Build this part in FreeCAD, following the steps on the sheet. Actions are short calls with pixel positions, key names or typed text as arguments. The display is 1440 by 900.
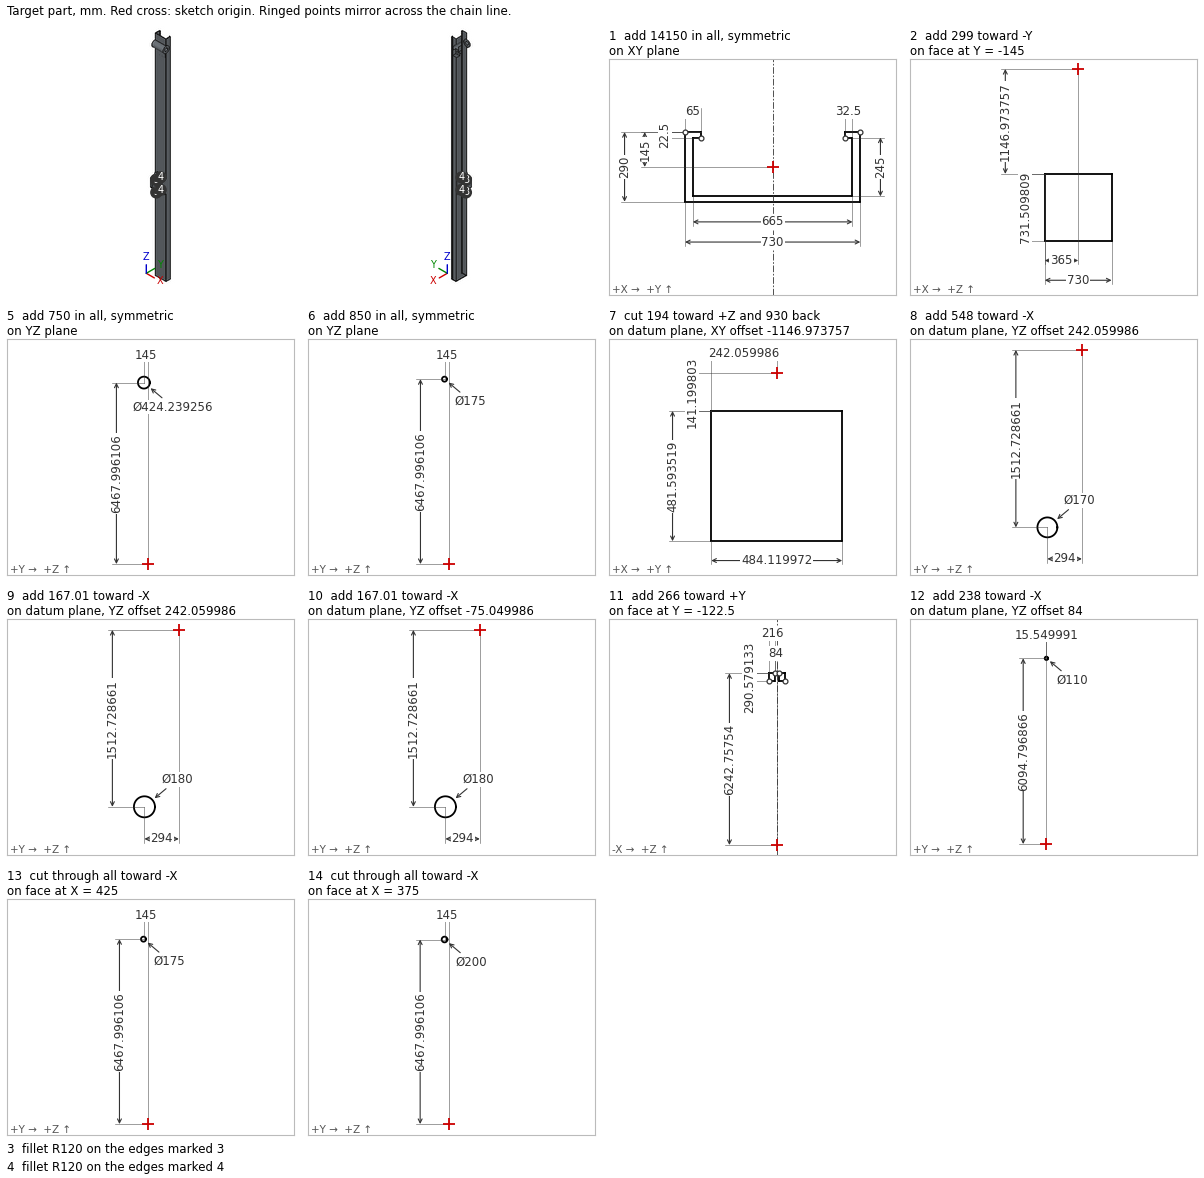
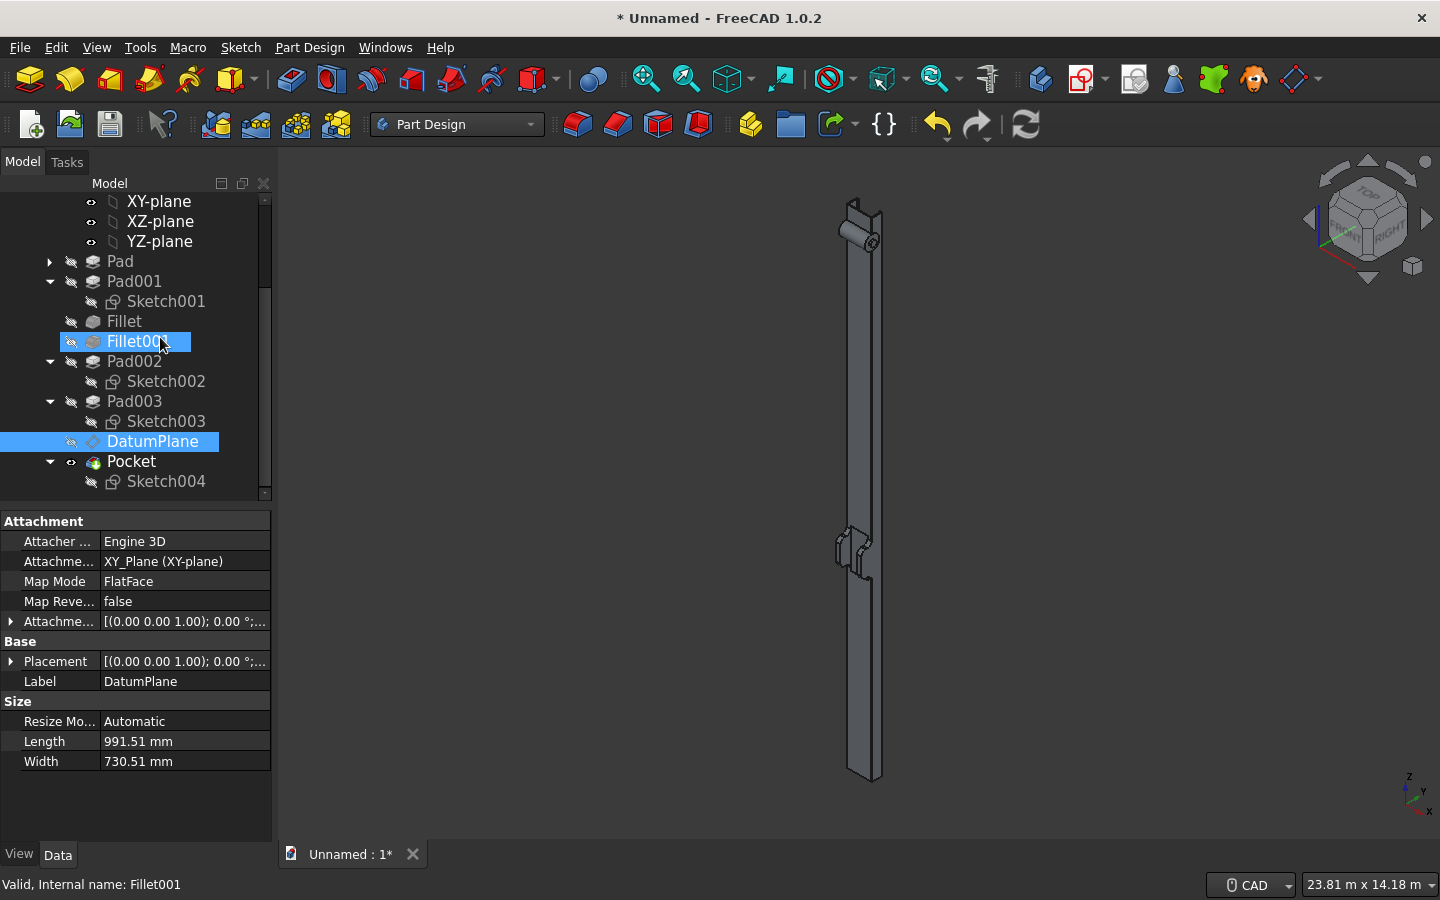
scroll(160, 337, up, 15)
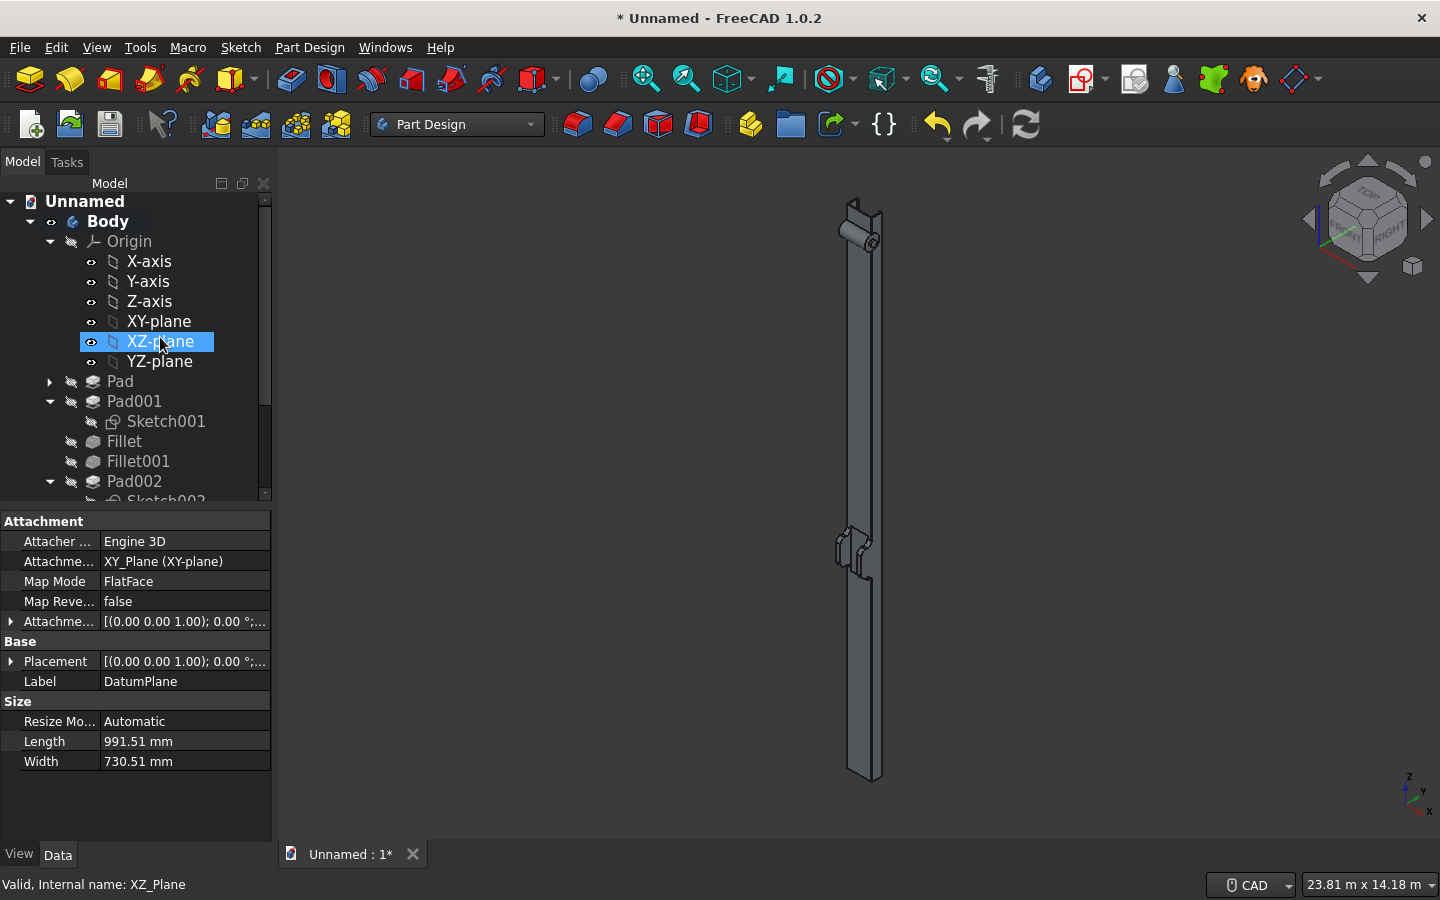
click(136, 362)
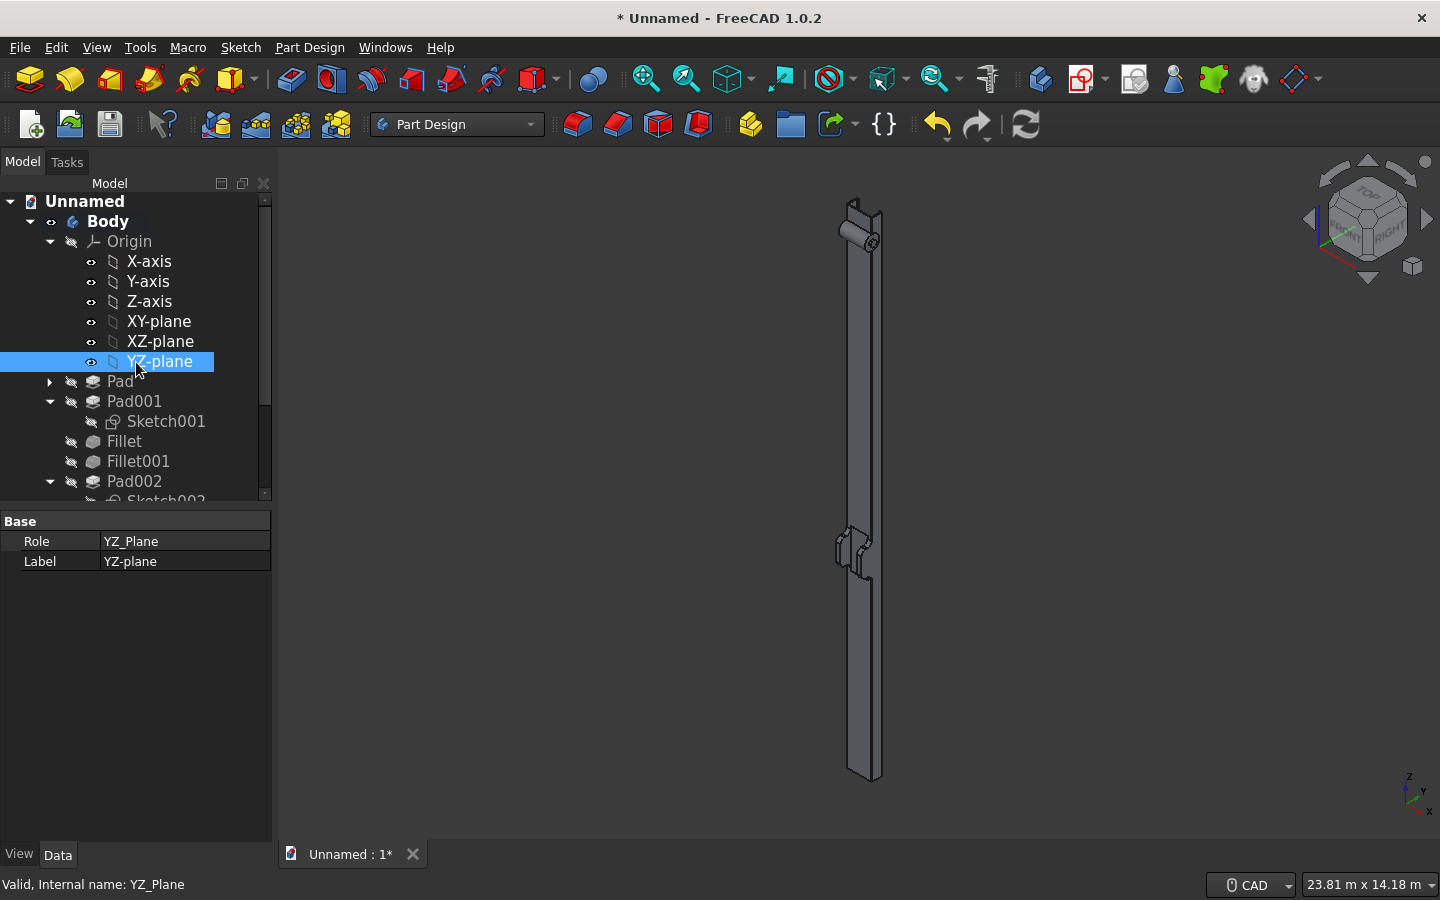
click(1294, 80)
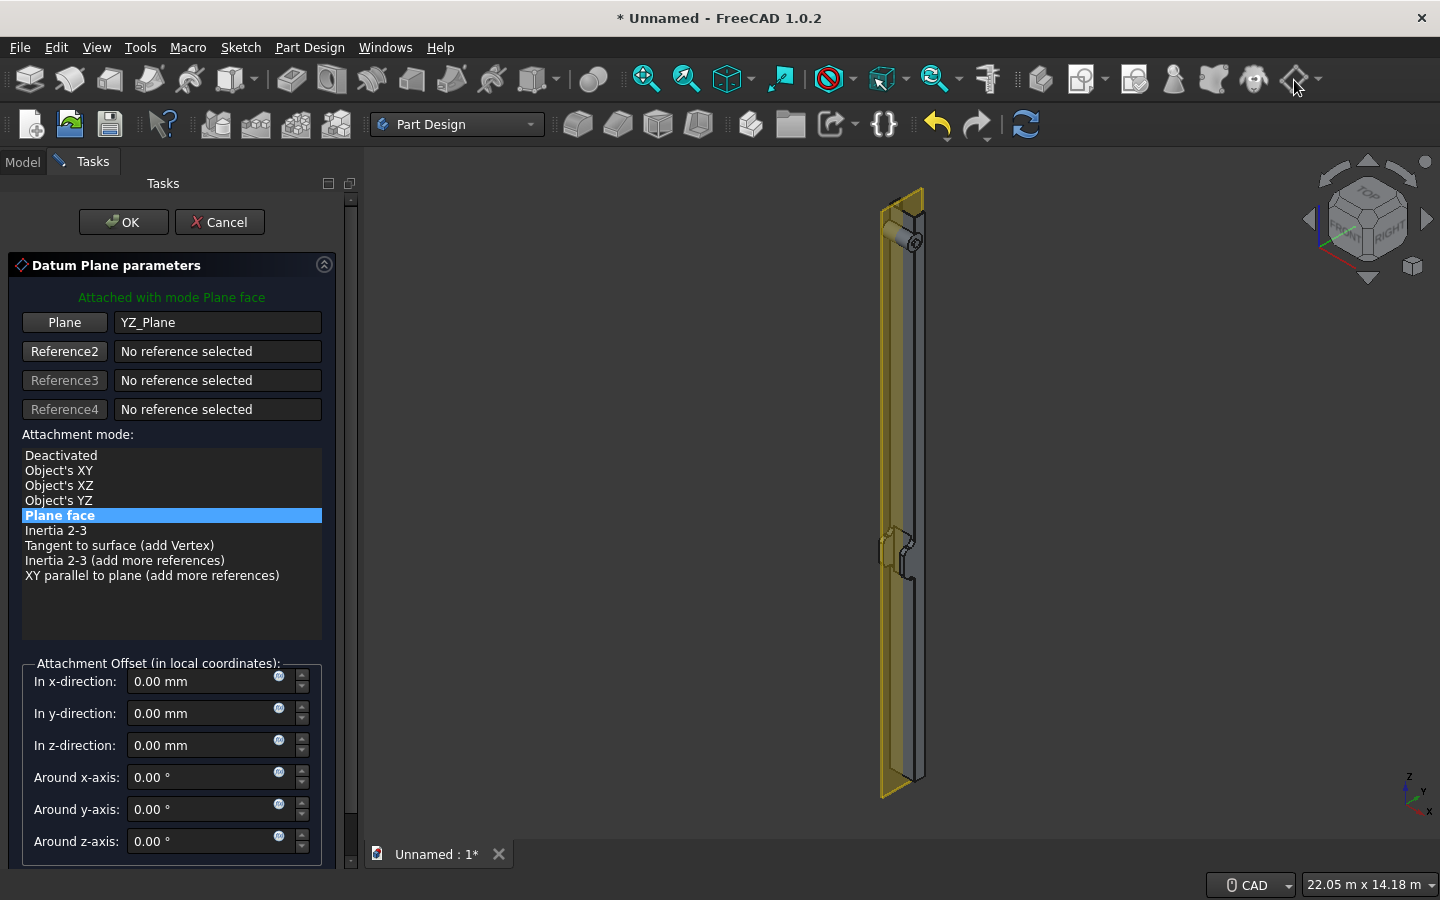
triple_click(210, 745)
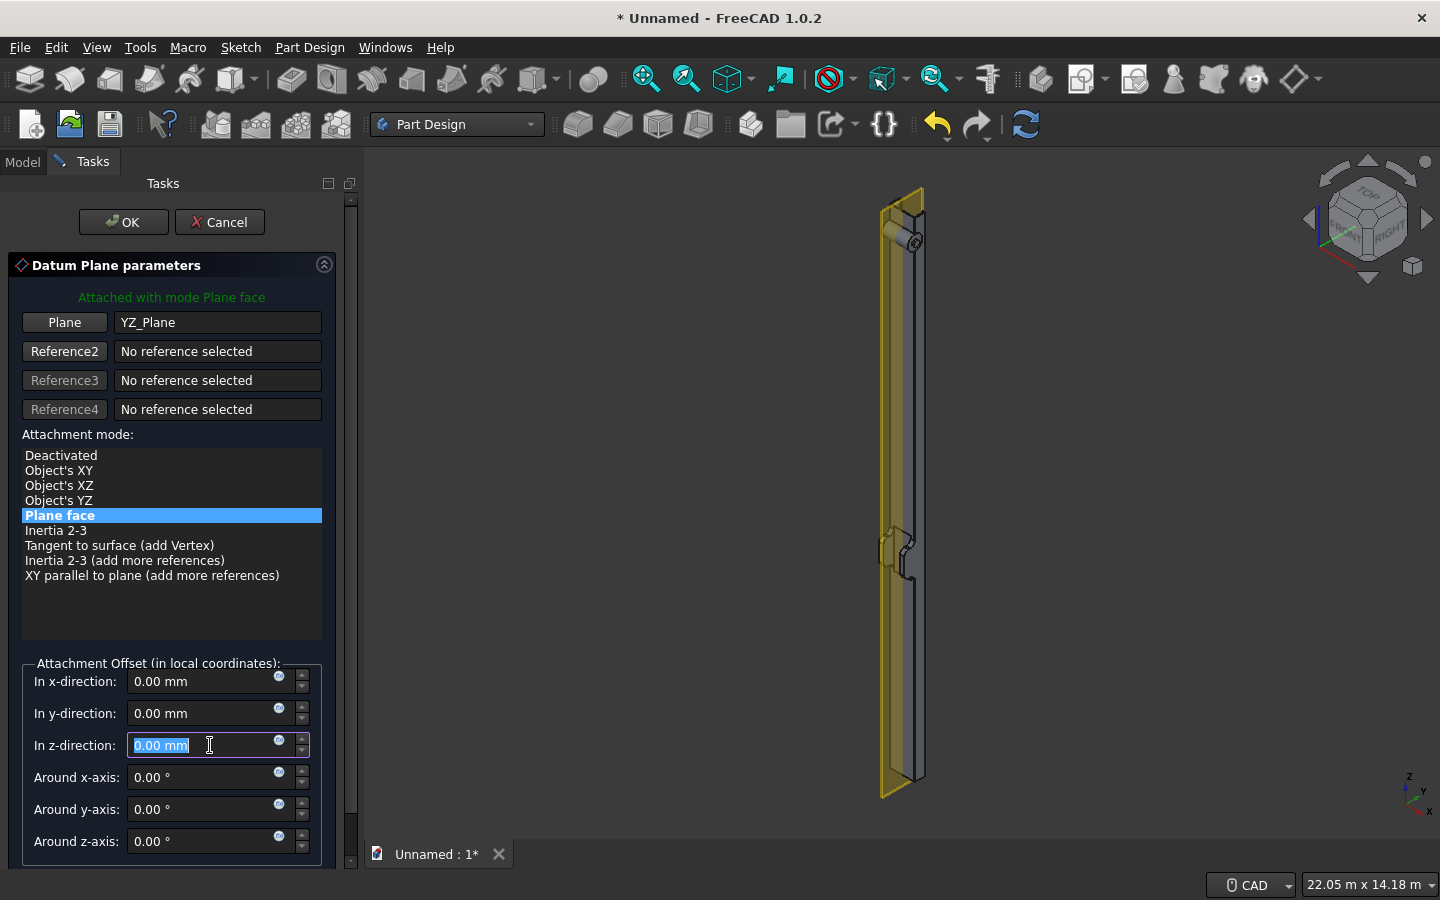
text(242.059986)
key(Tab)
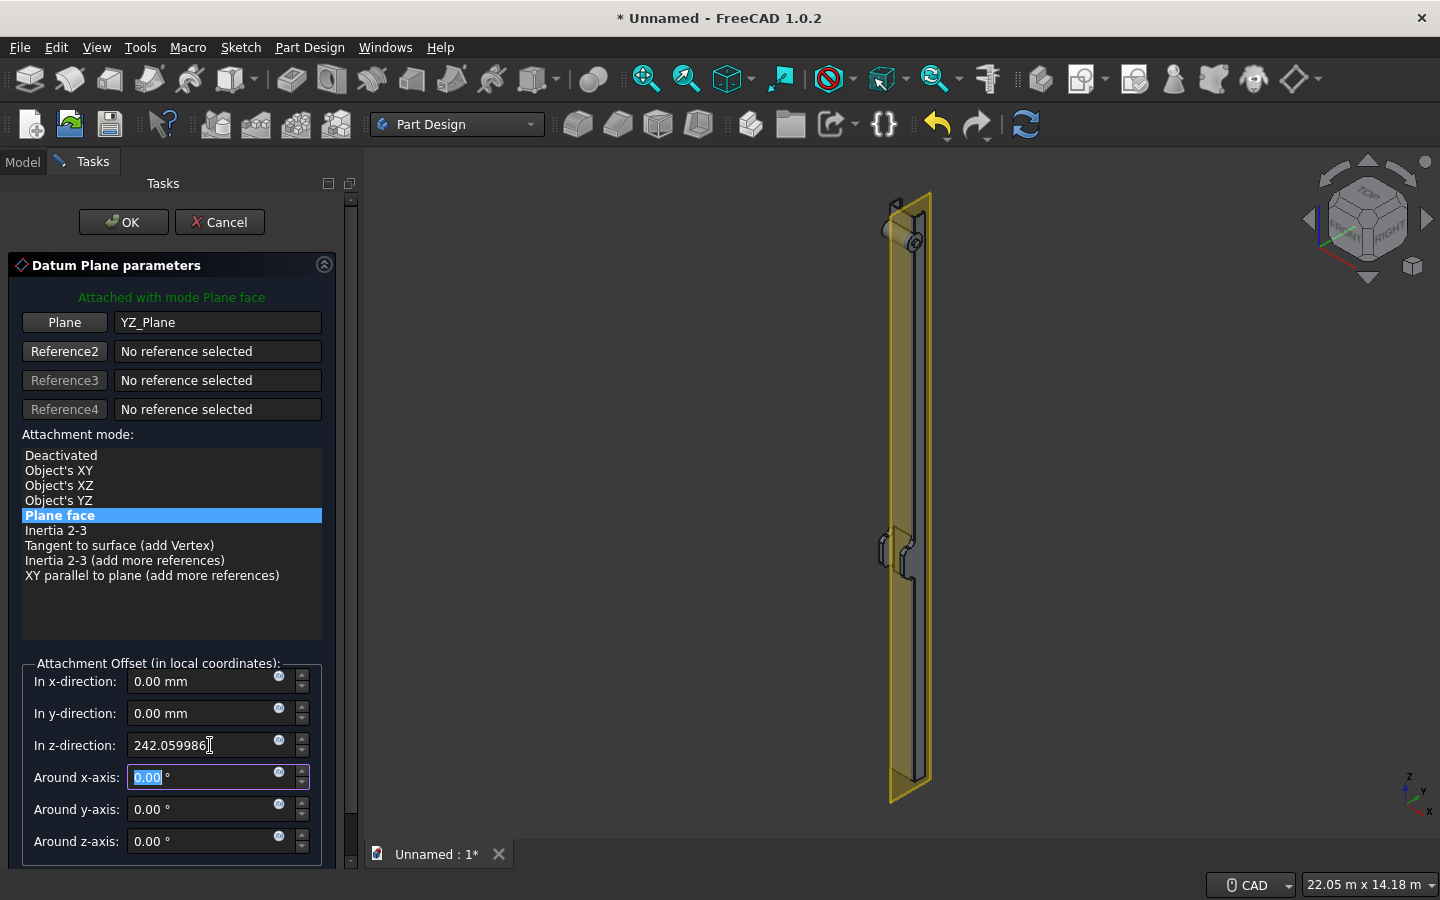
click(124, 222)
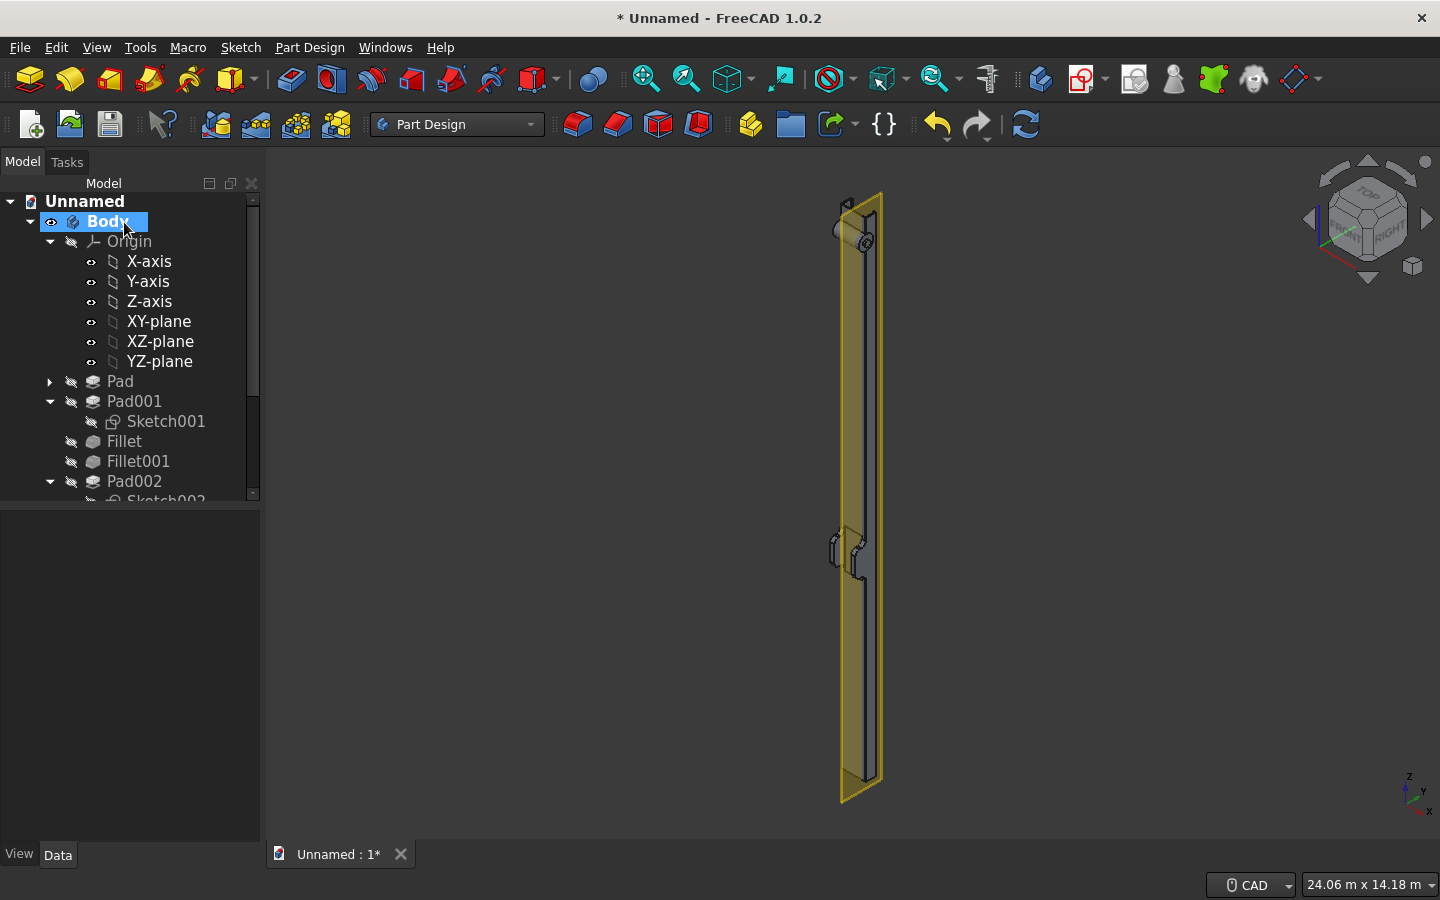
scroll(100, 337, down, 3)